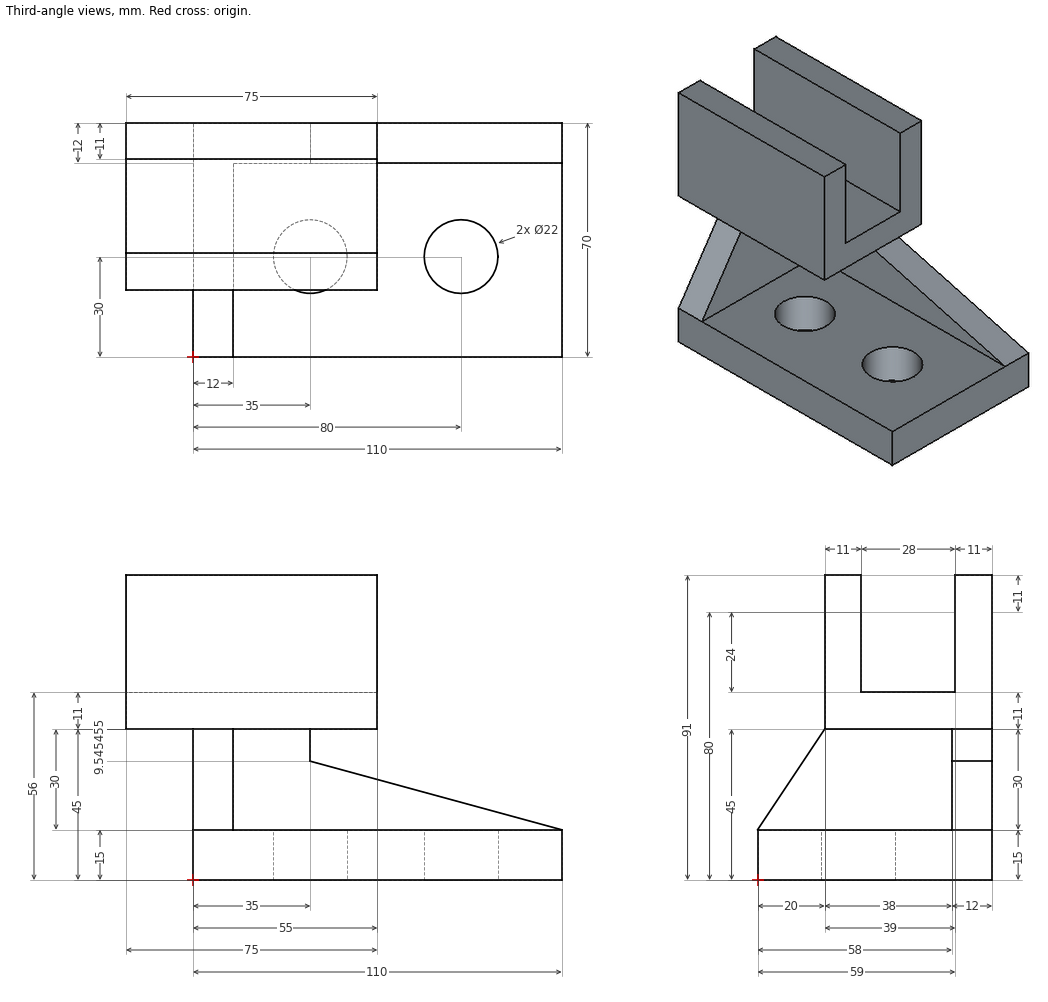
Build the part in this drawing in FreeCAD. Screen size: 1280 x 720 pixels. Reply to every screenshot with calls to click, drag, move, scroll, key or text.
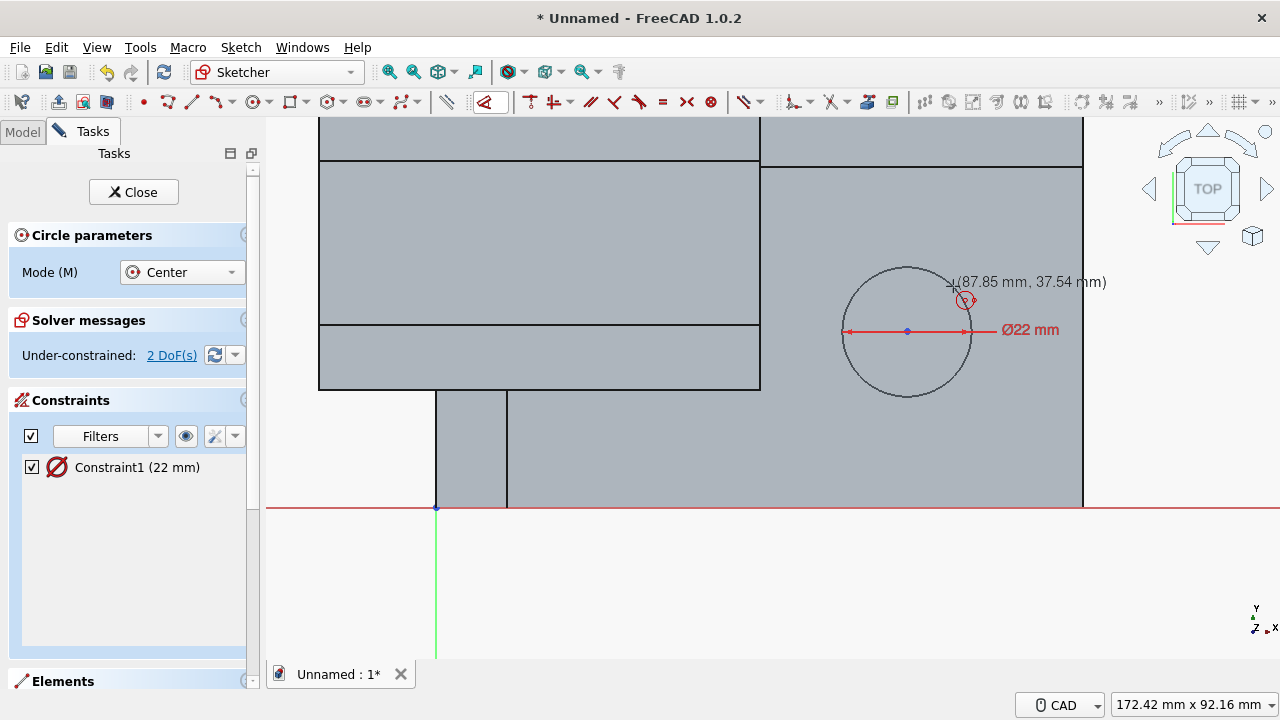
click(642, 331)
move(688, 286)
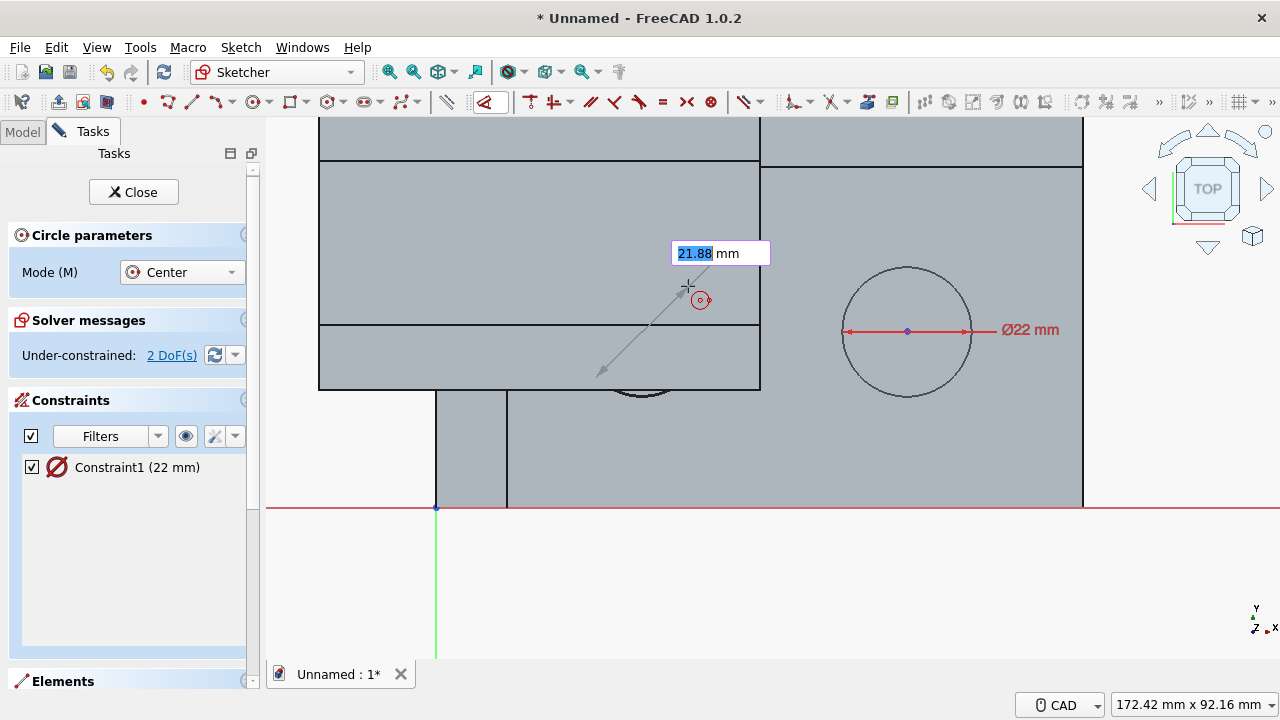
text(22)
key(Return)
key(Escape)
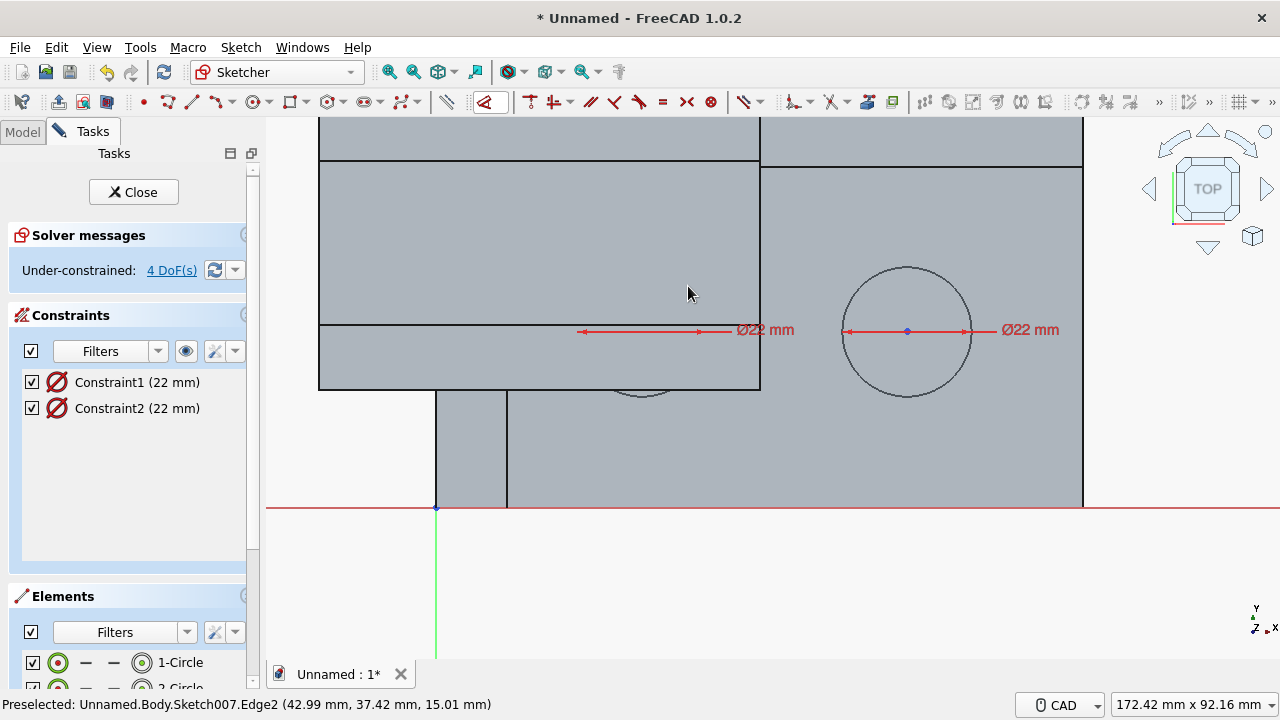
click(907, 332)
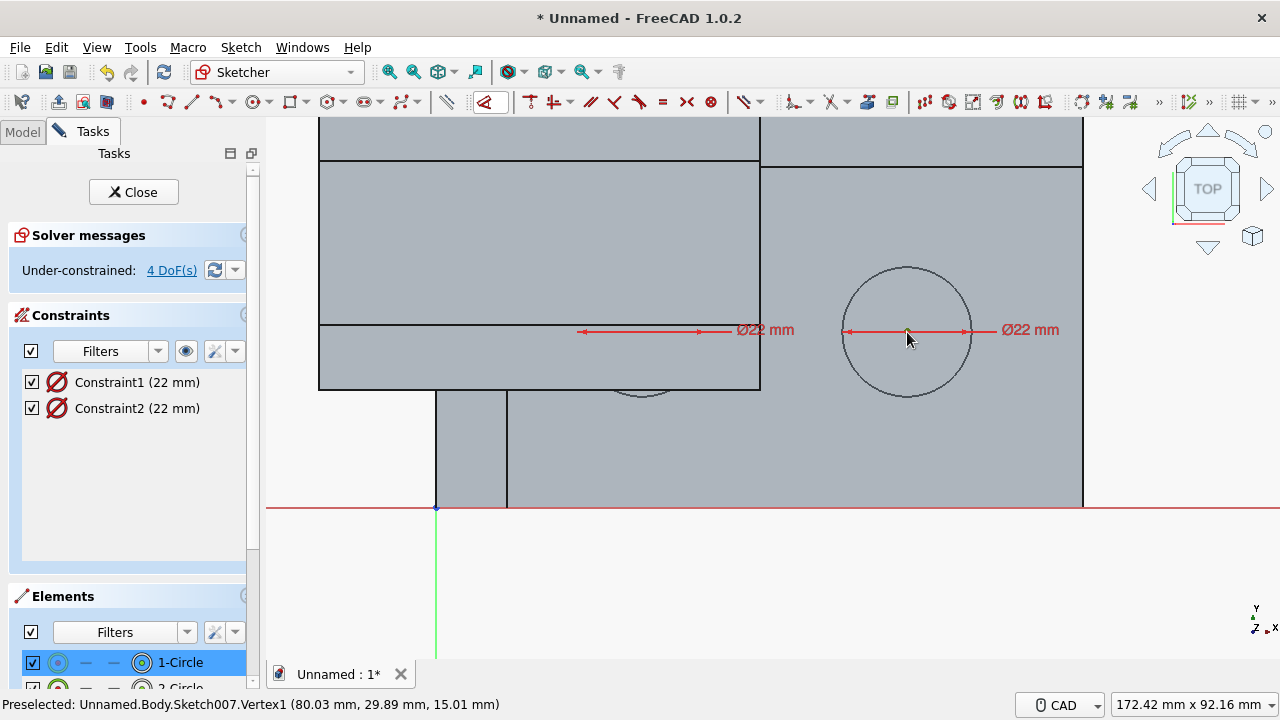
click(642, 332)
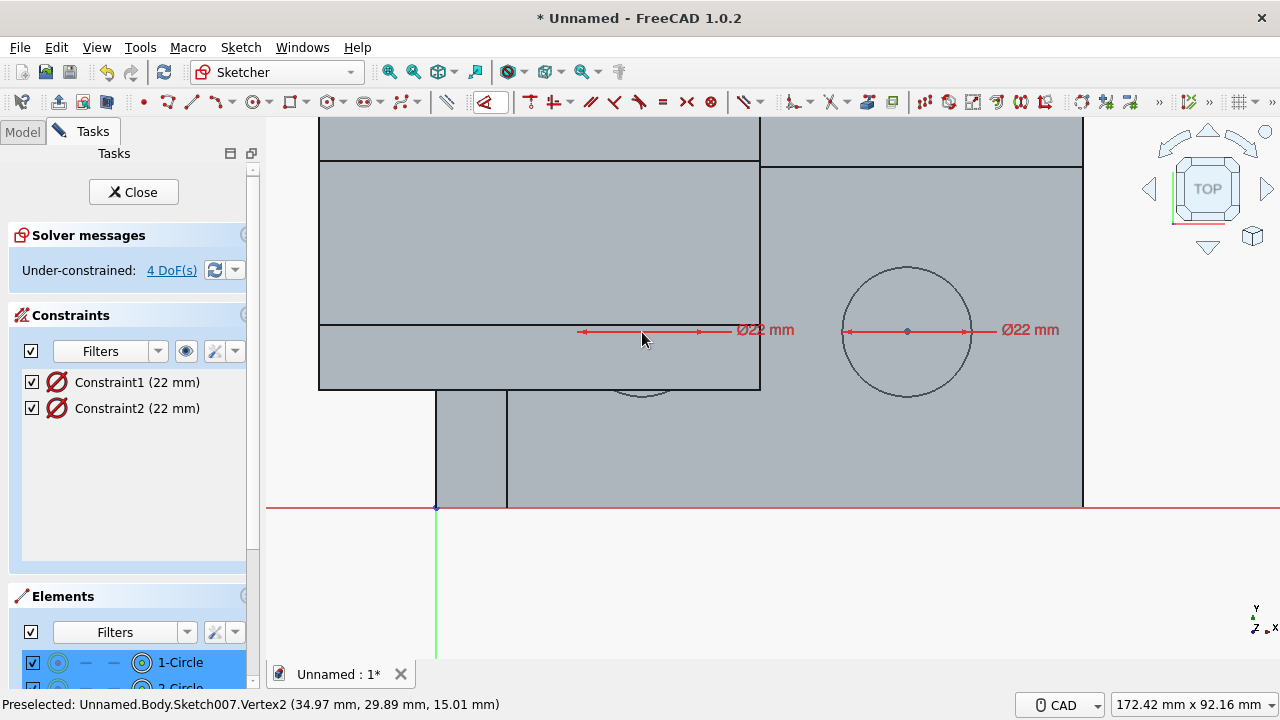
key(h)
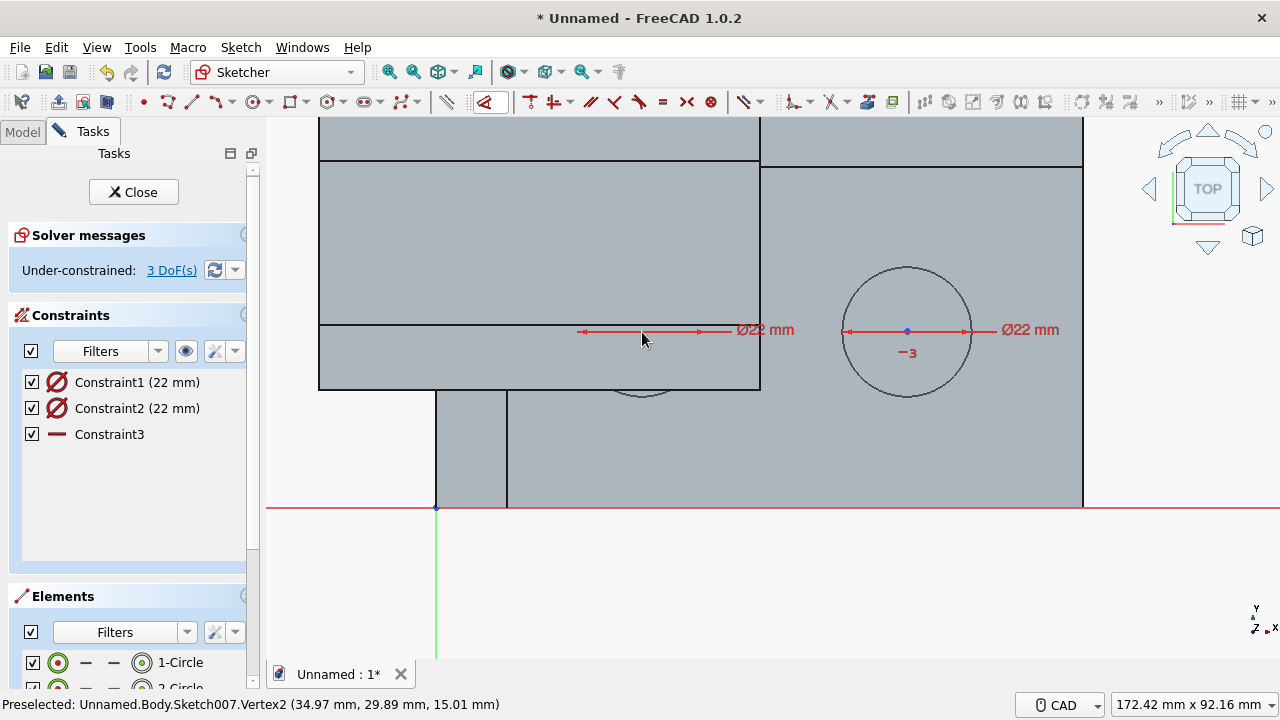
click(907, 332)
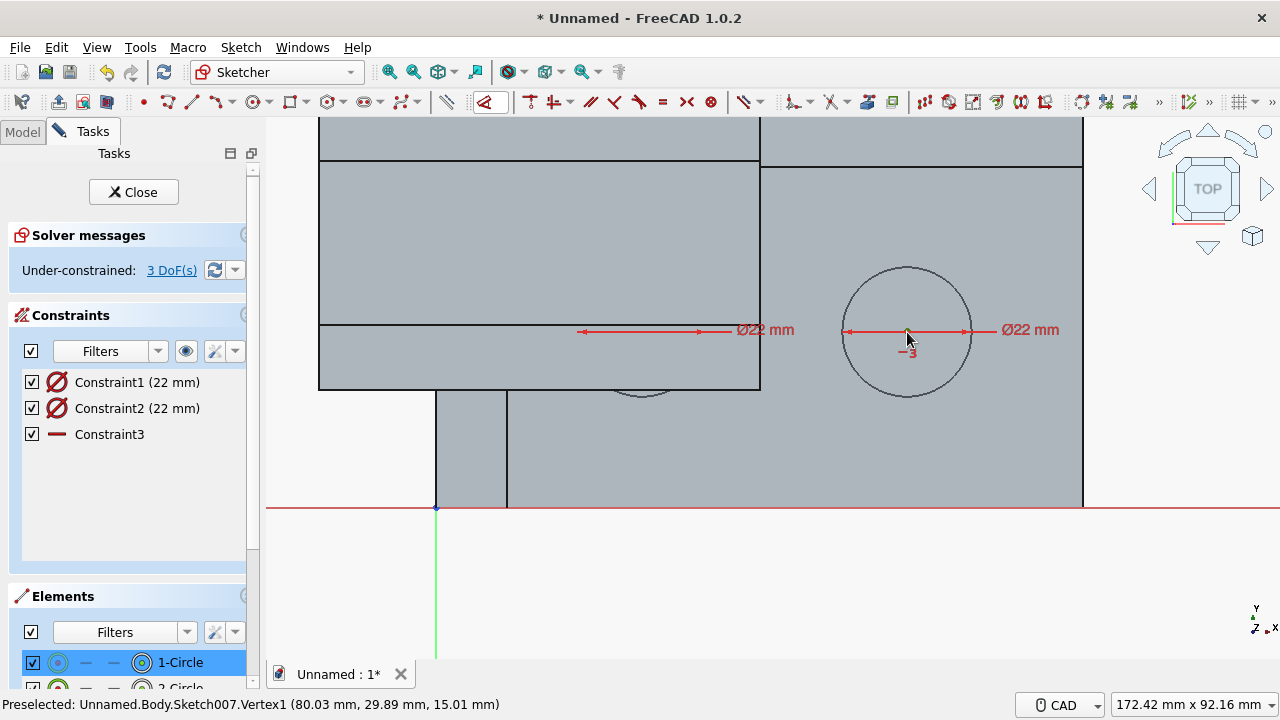
key(l)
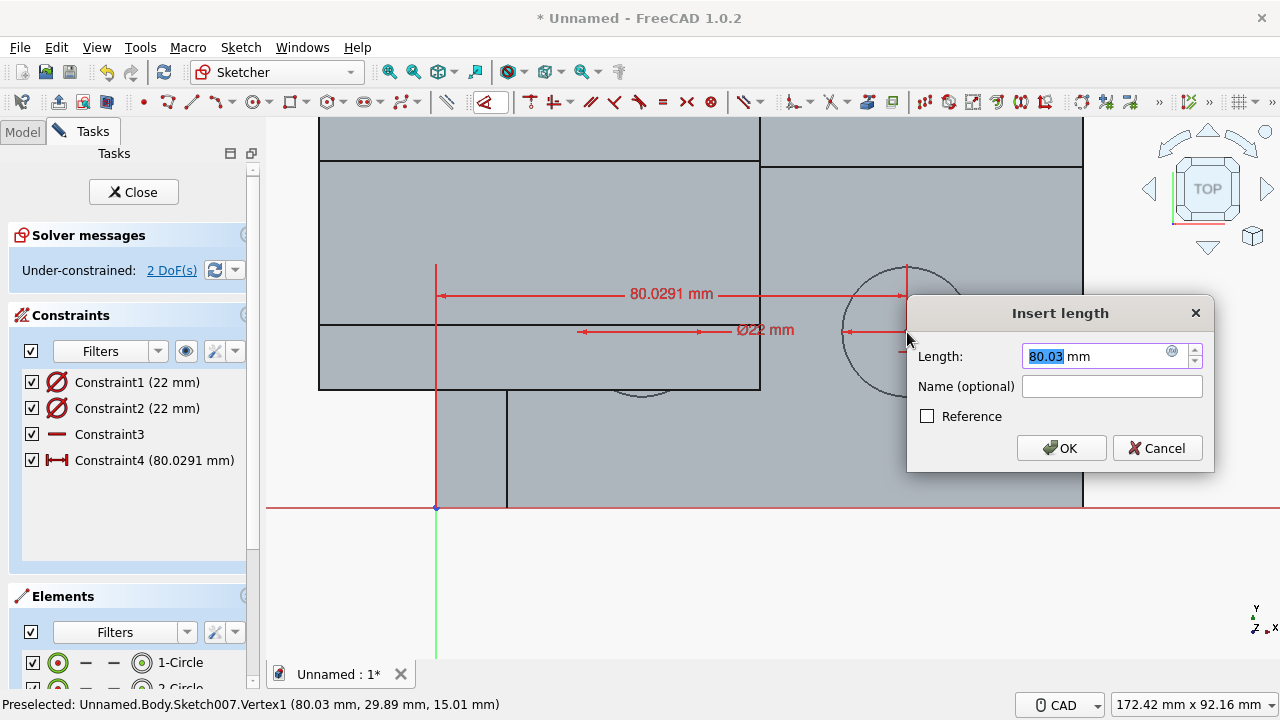
text(80)
key(Return)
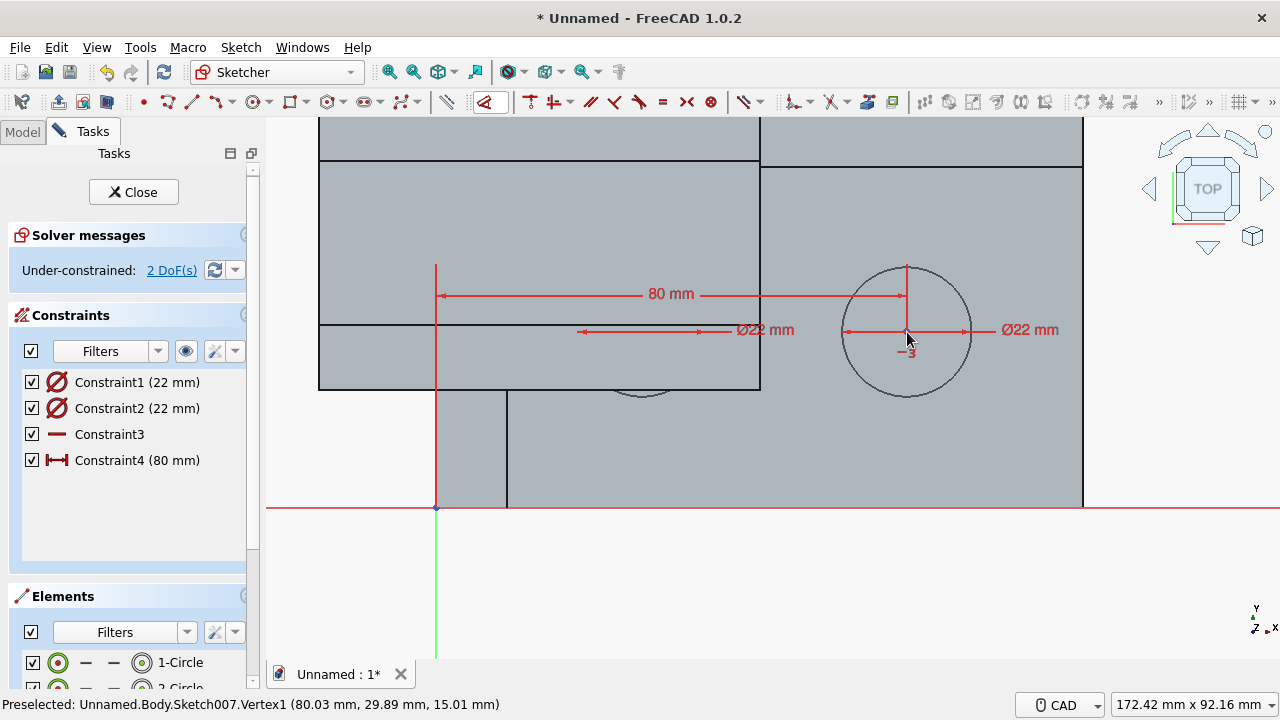
click(907, 332)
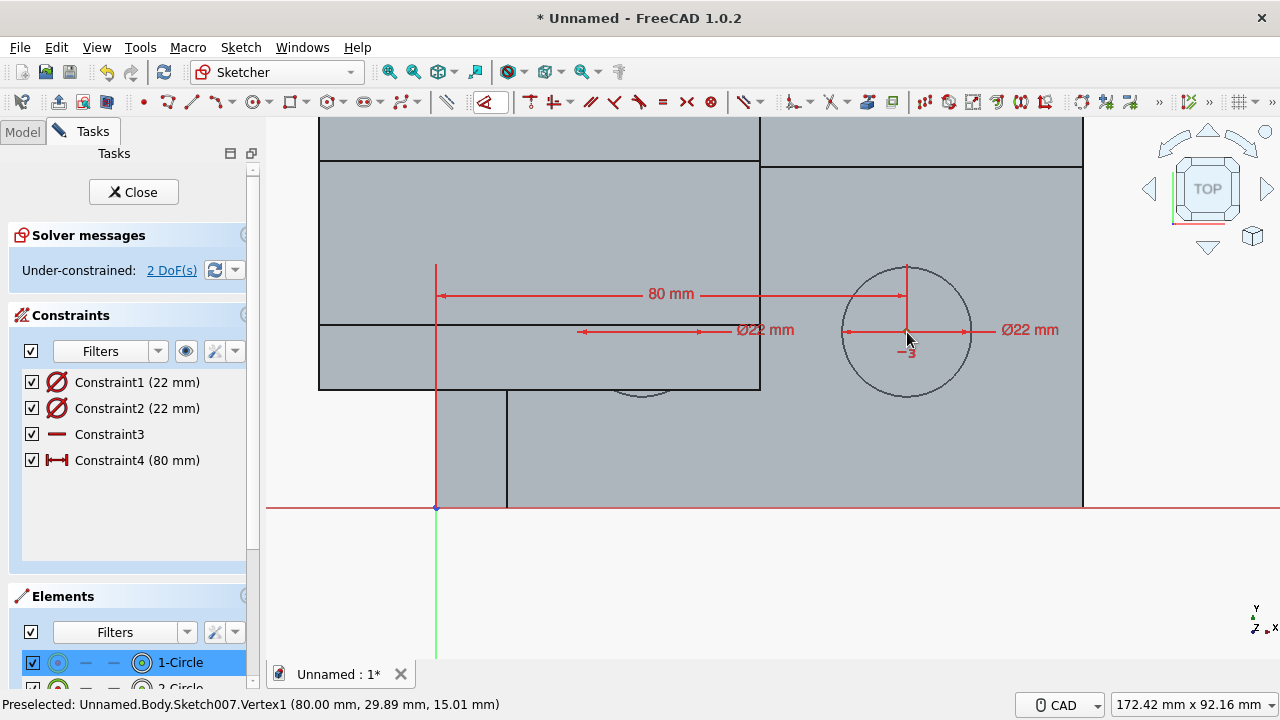
key(i)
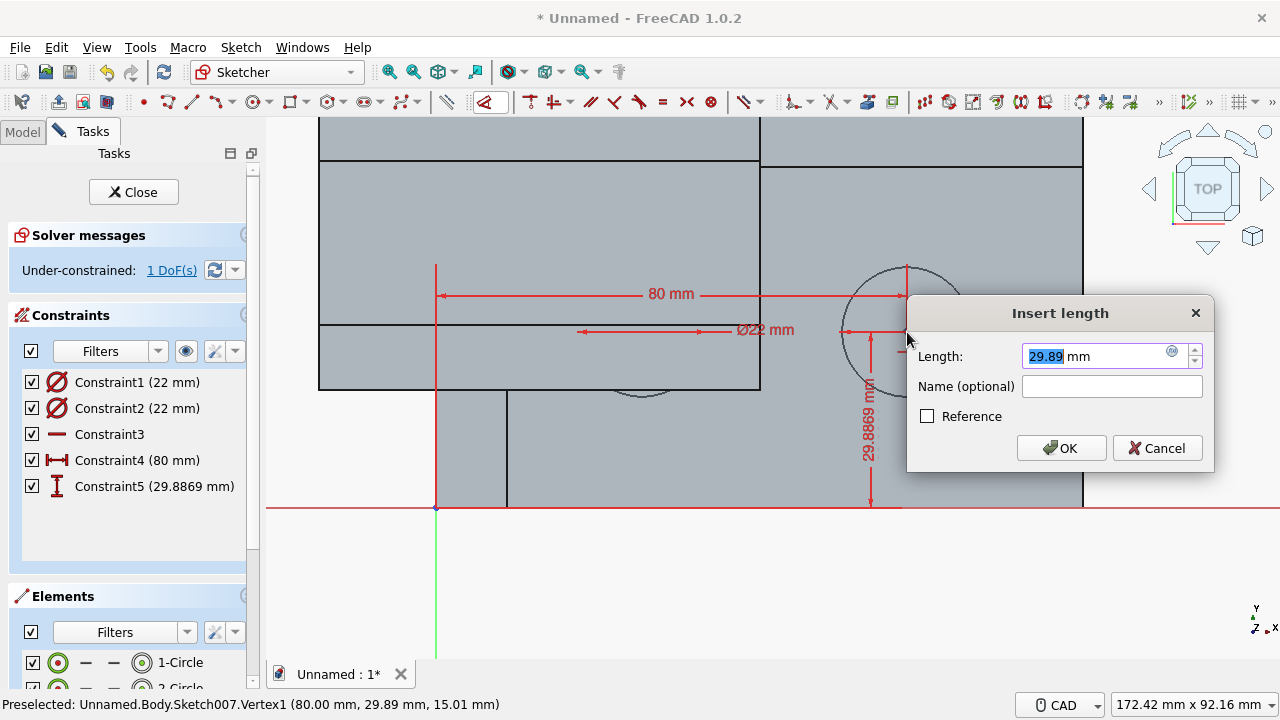
text(30)
key(Return)